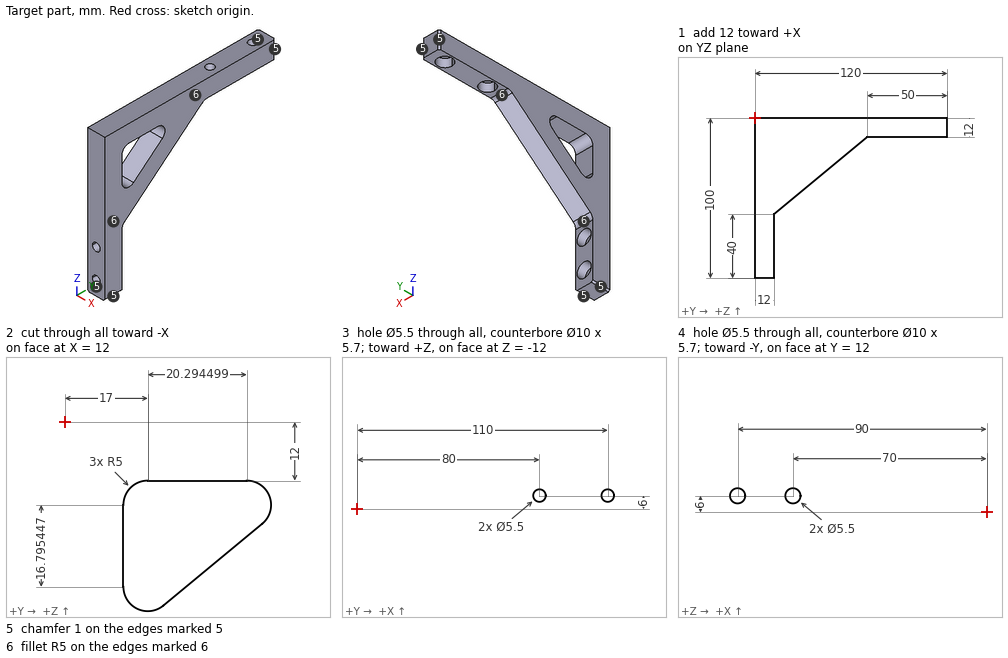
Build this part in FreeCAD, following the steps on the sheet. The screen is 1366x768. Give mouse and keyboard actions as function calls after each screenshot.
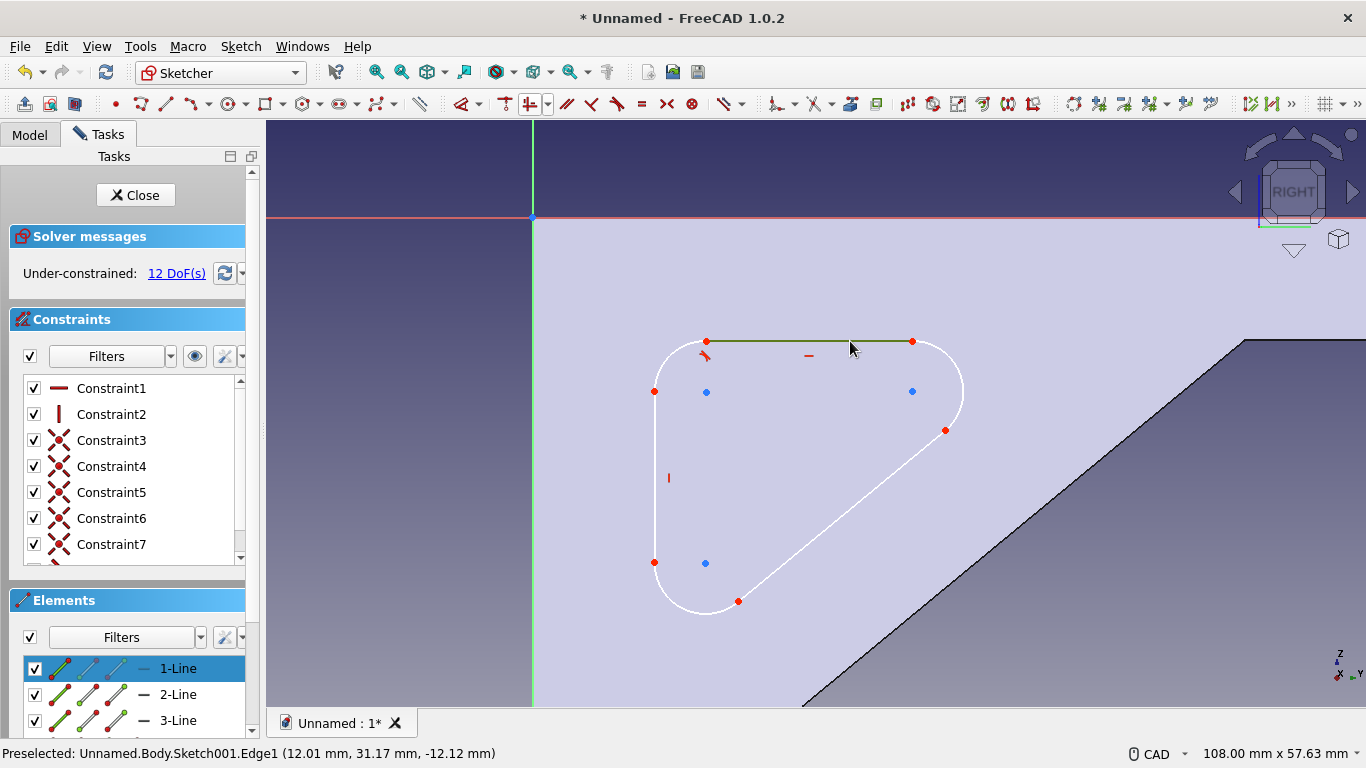
click(963, 399)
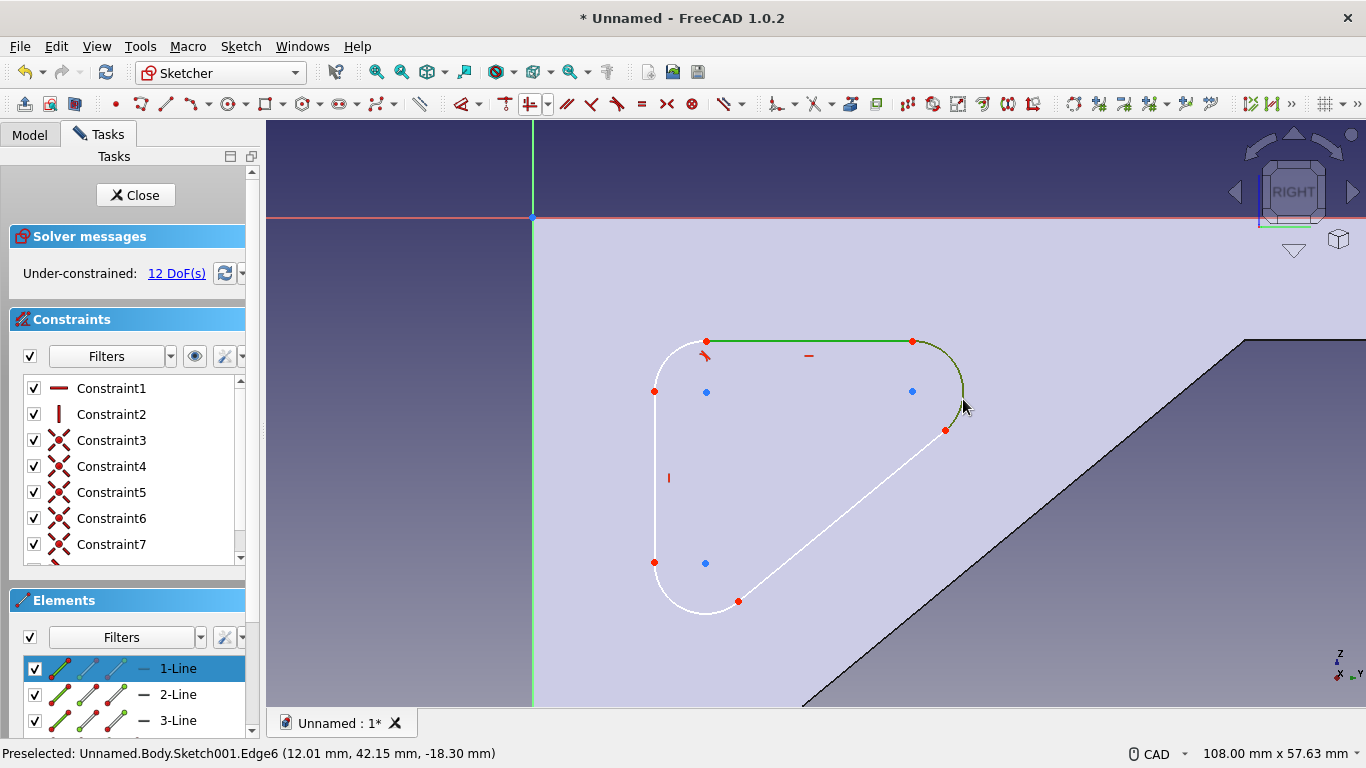
click(617, 104)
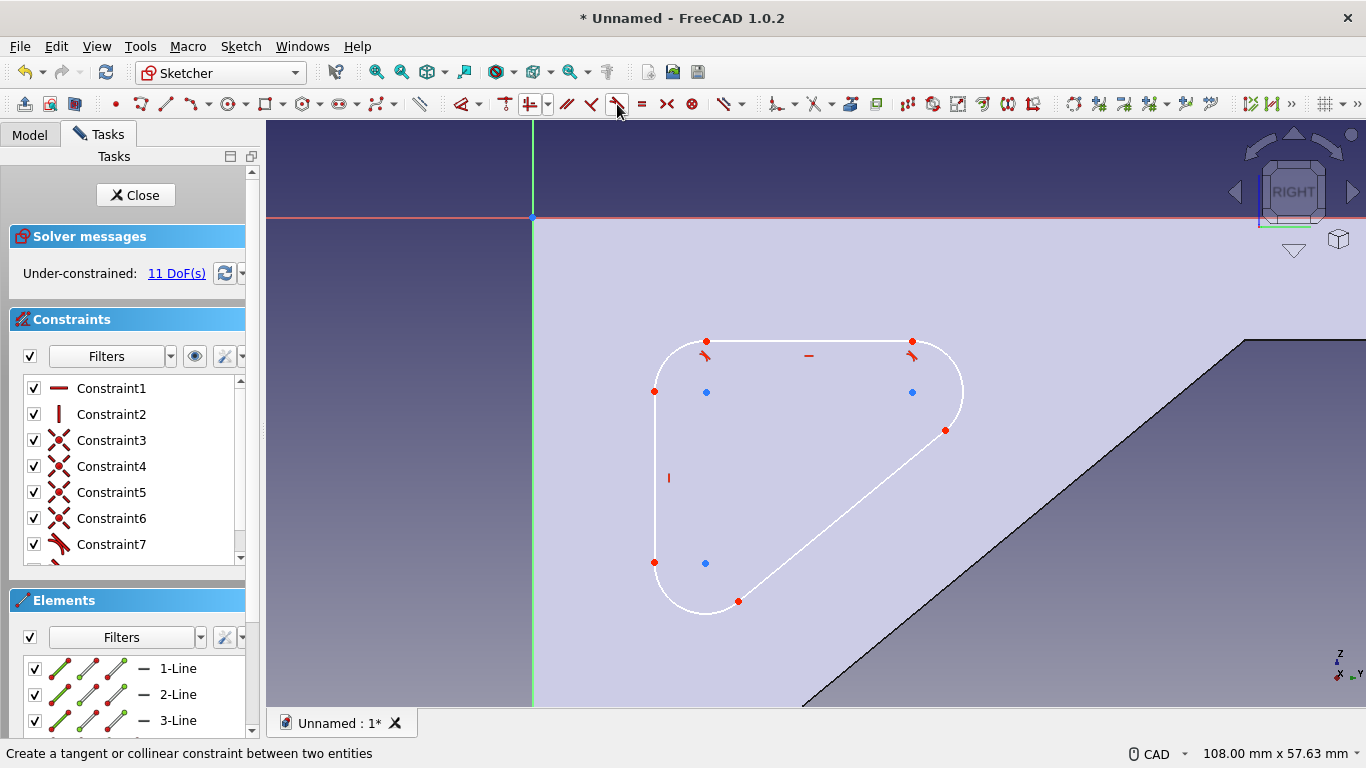
click(655, 443)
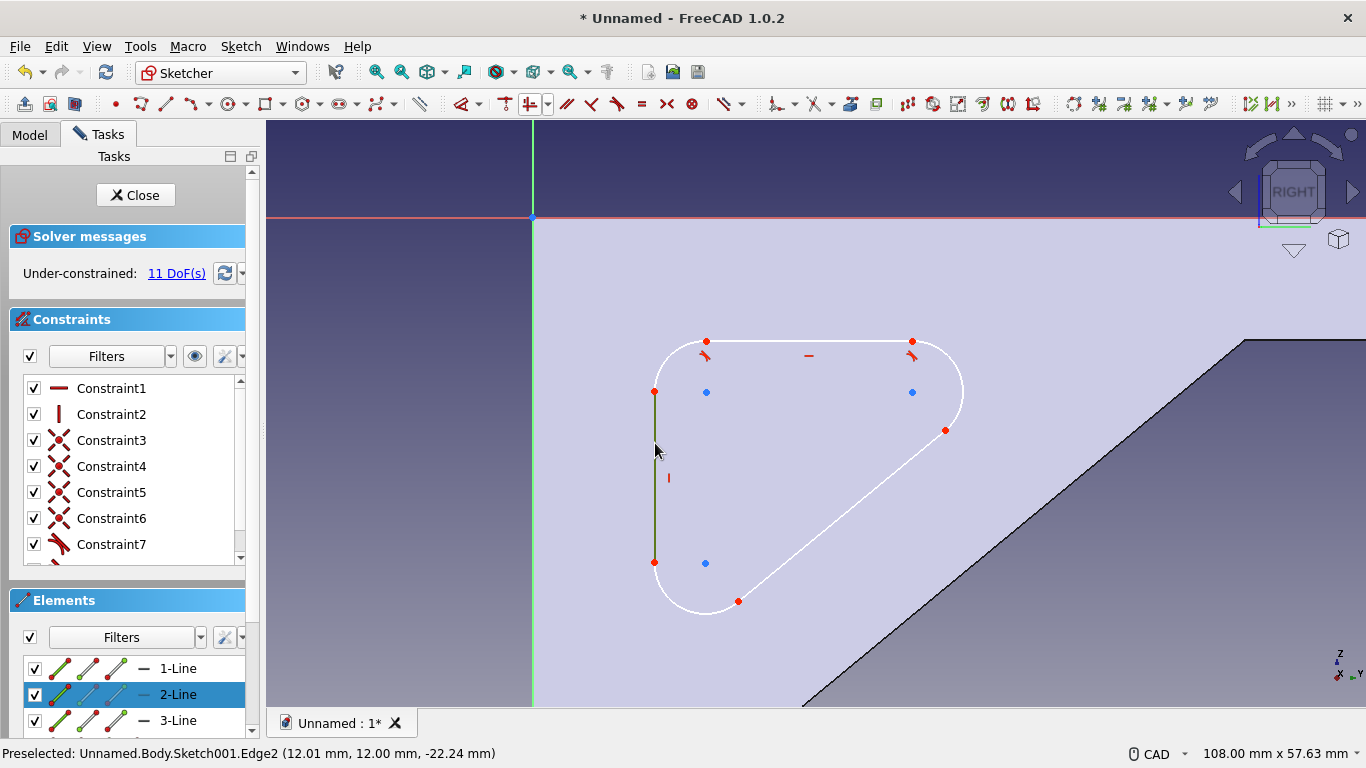
click(683, 347)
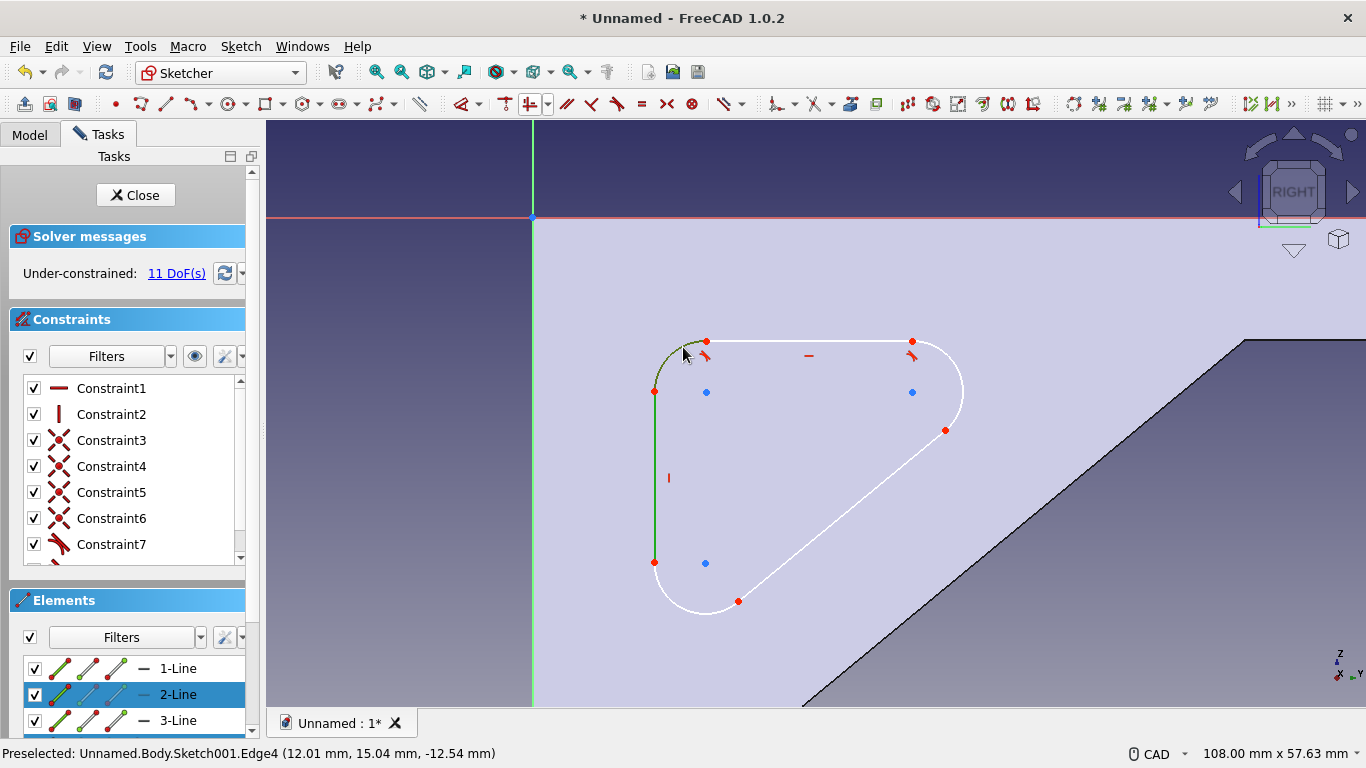
click(617, 104)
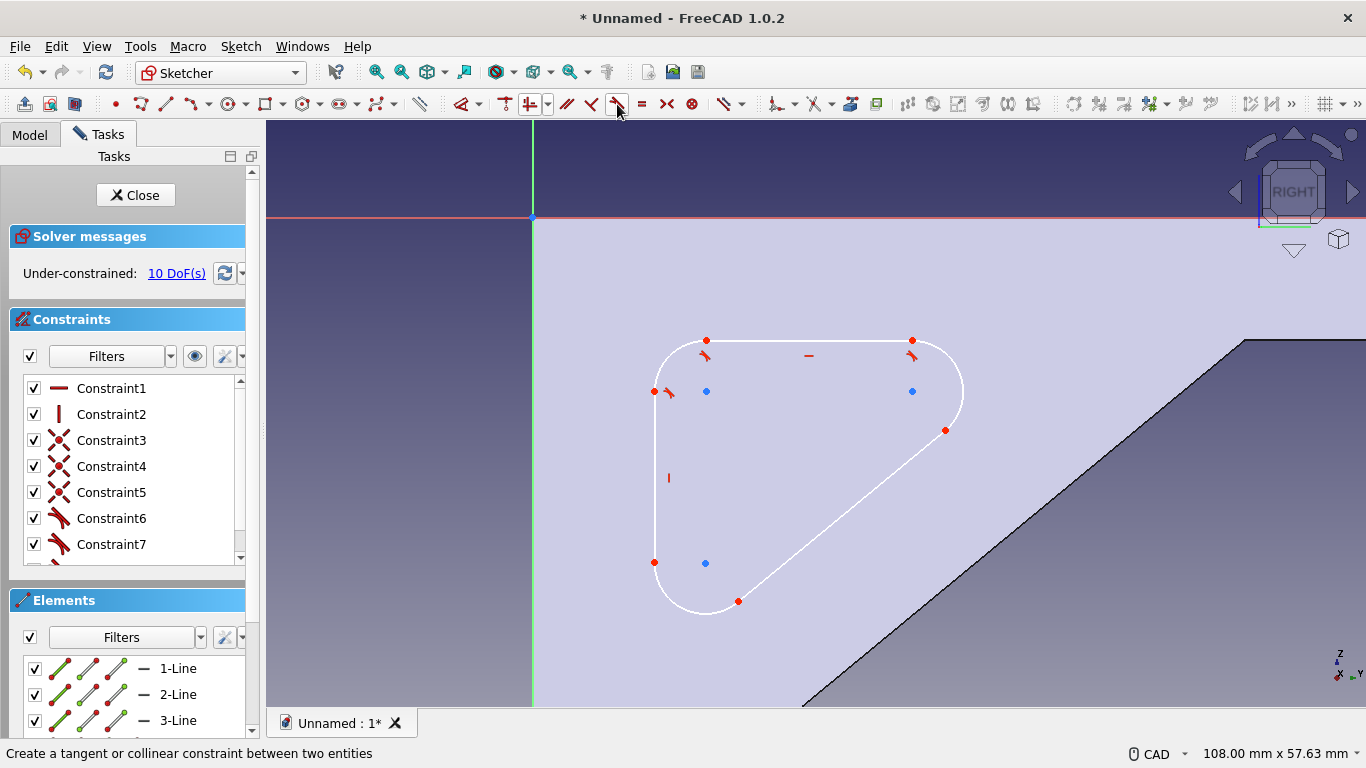
click(655, 443)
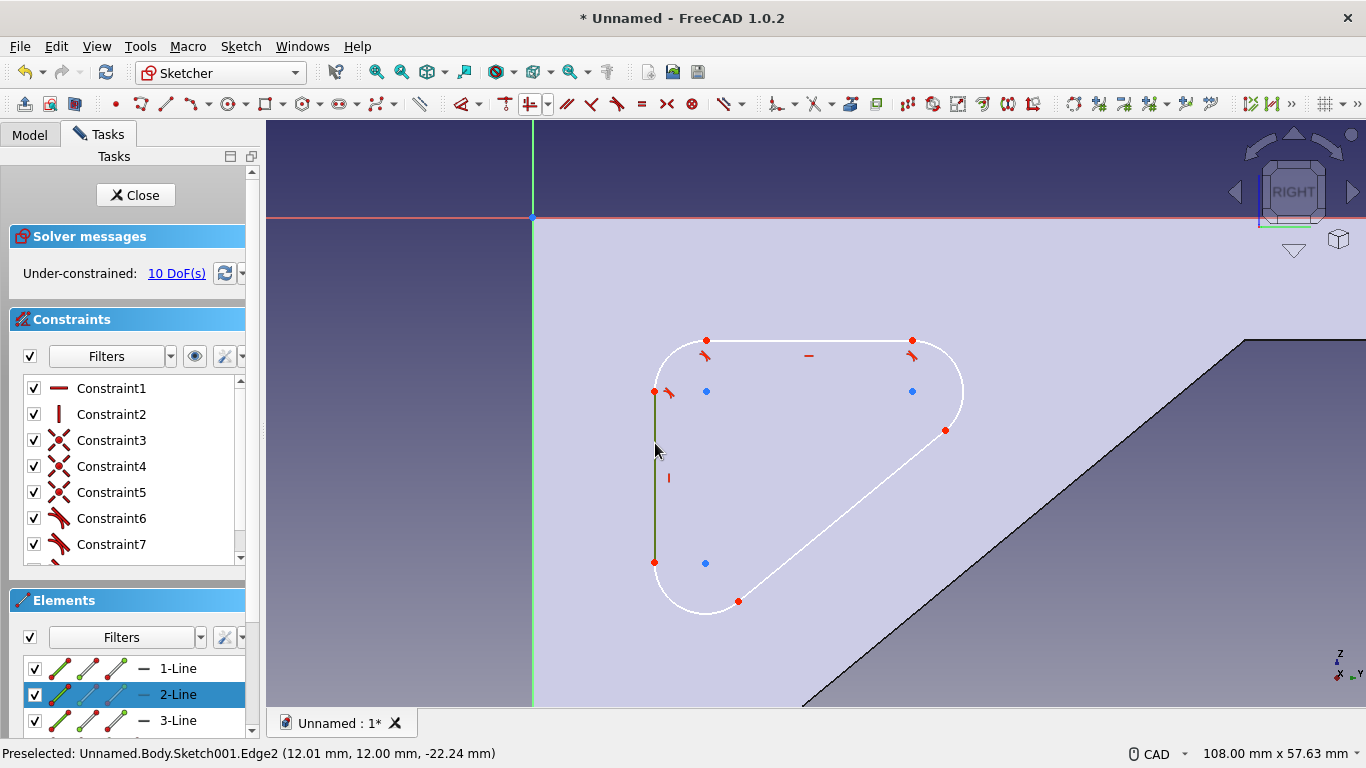
click(666, 595)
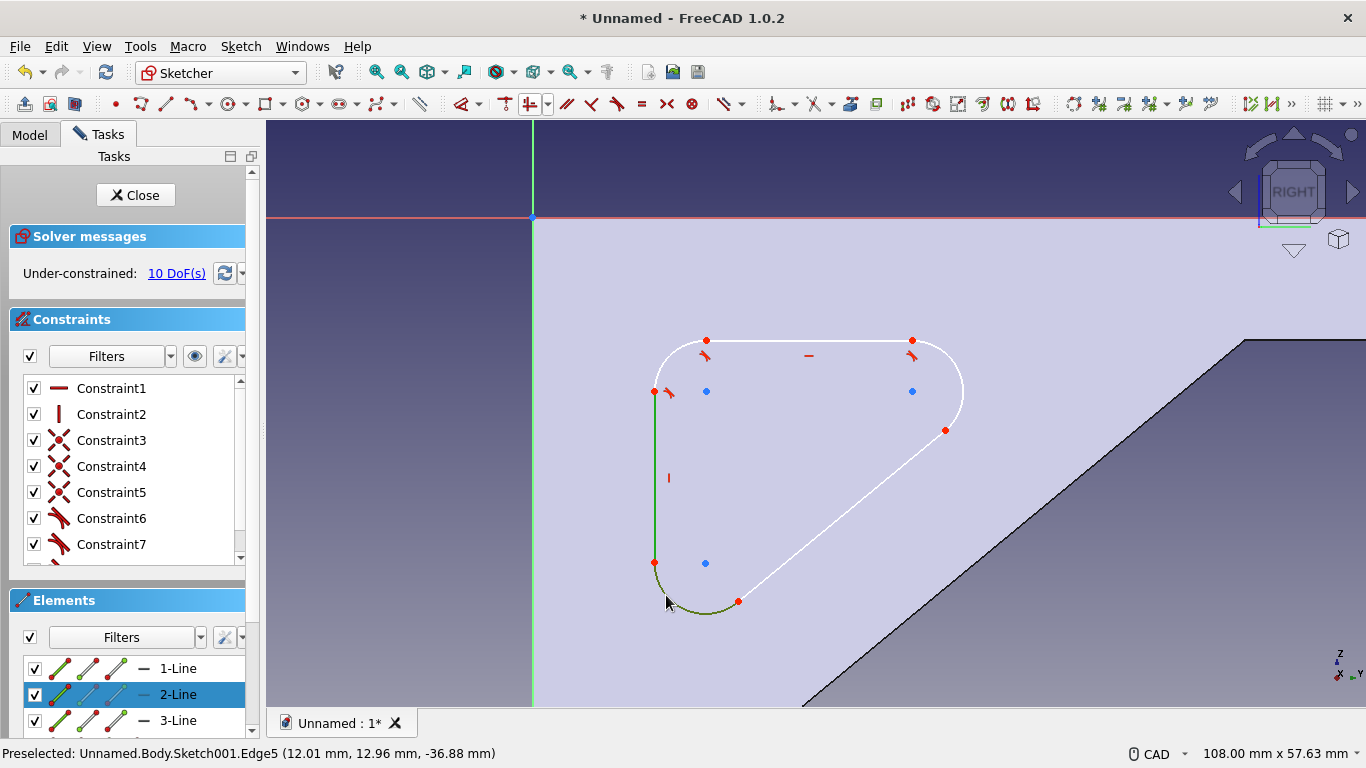
click(617, 104)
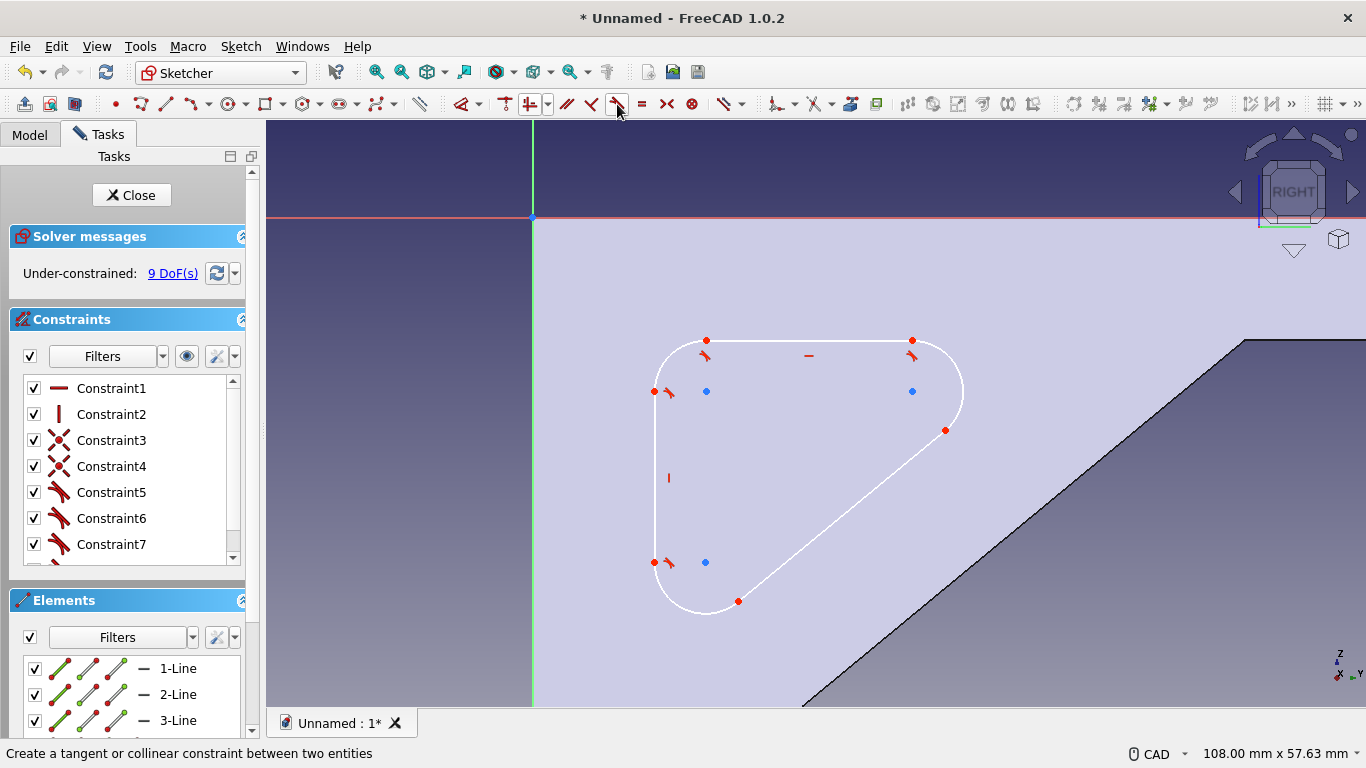
click(800, 551)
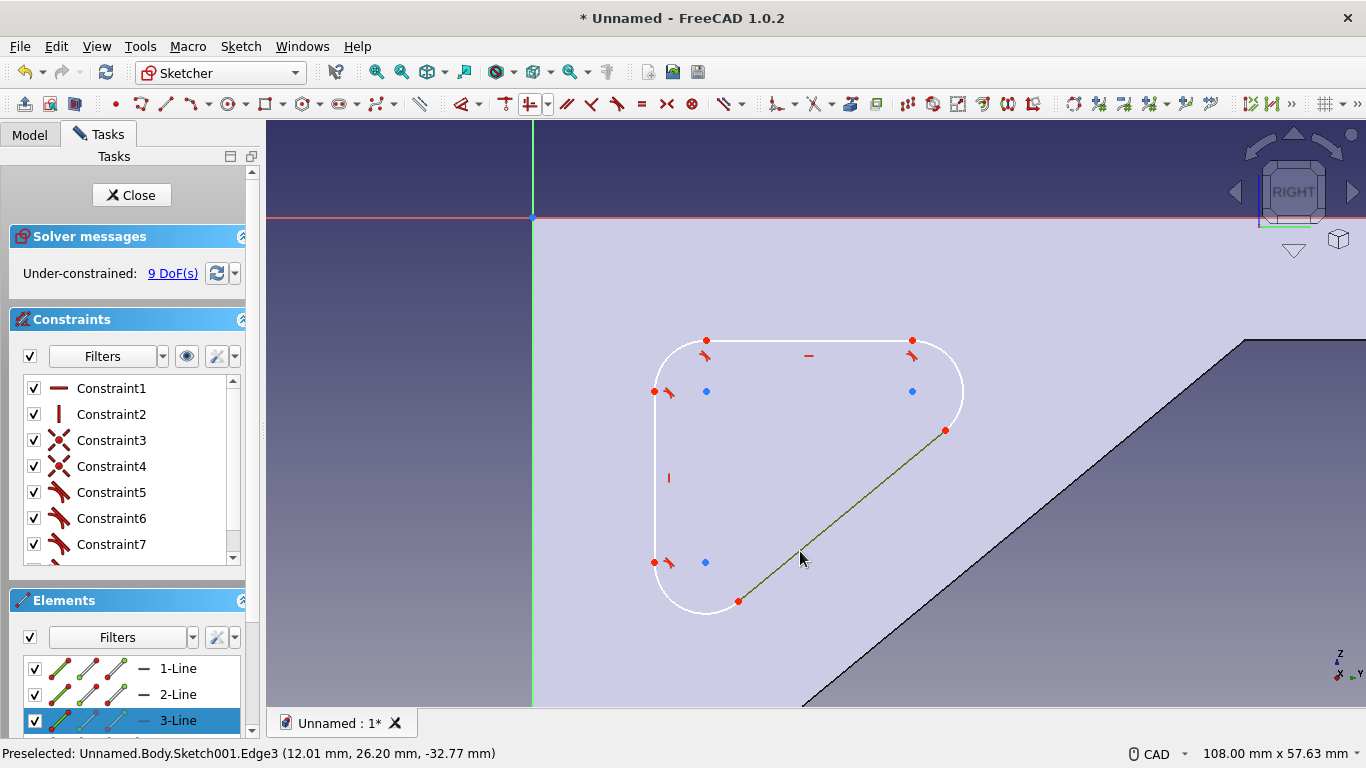
click(666, 595)